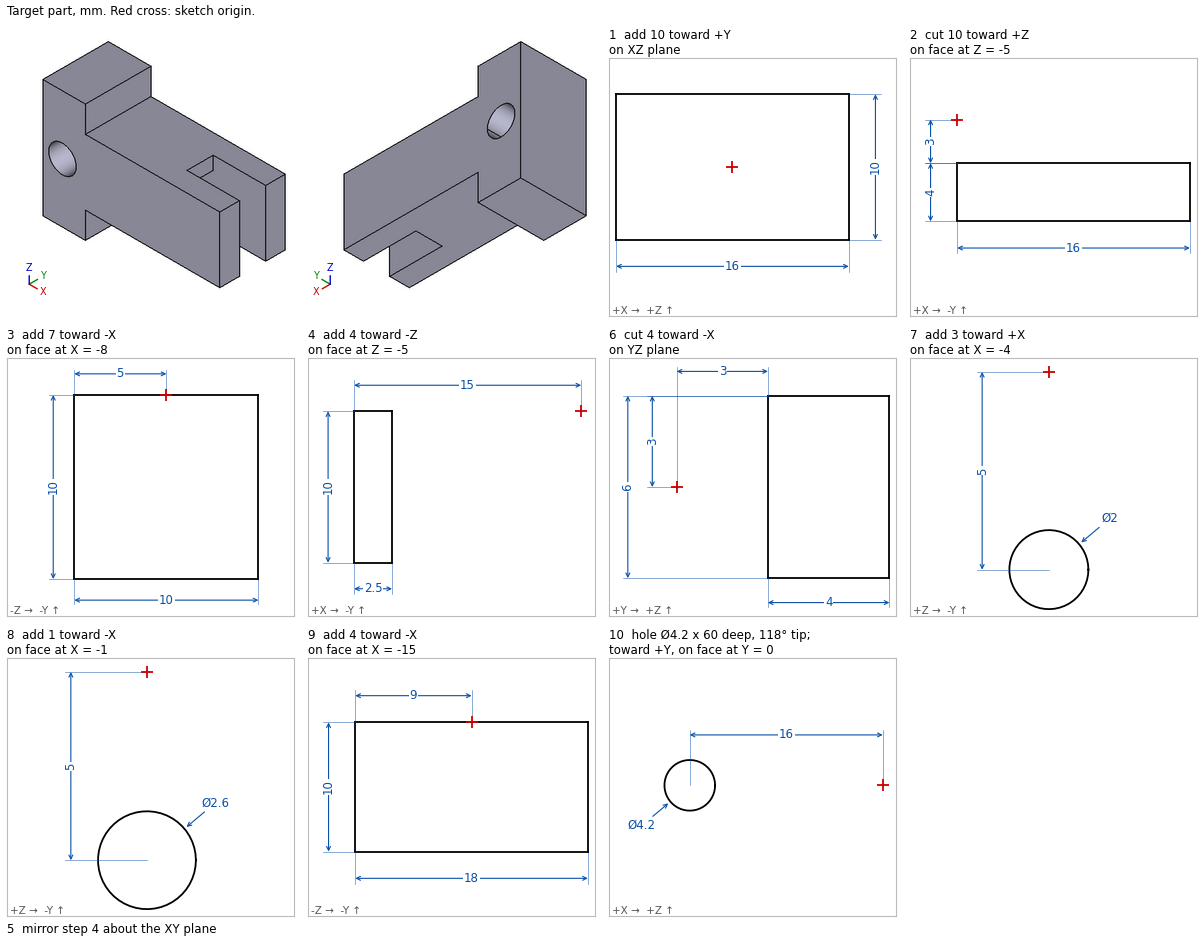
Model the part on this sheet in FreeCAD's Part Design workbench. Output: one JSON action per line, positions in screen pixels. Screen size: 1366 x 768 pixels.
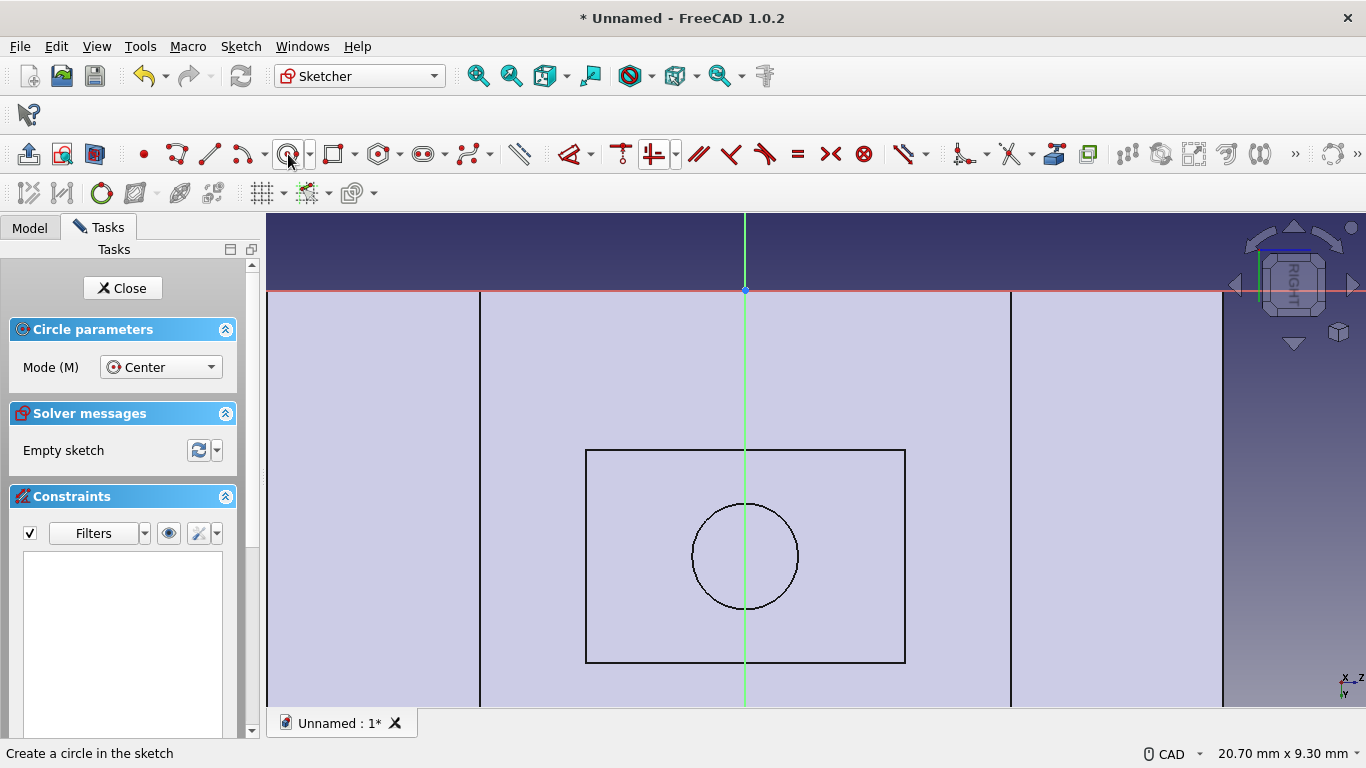
{"action": "left_click", "coordinate": [745, 556]}
{"action": "left_click", "coordinate": [794, 508]}
{"action": "key", "text": "Escape"}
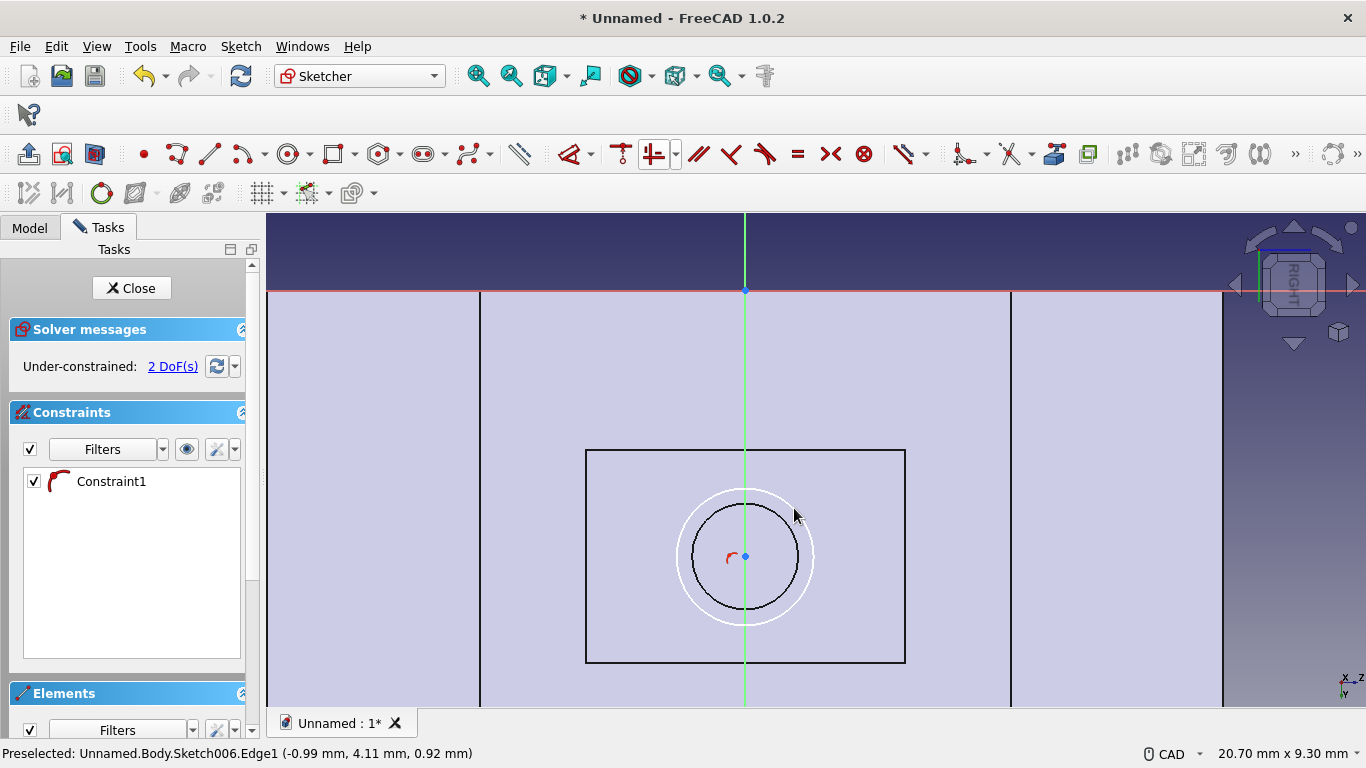
{"action": "left_click", "coordinate": [568, 154]}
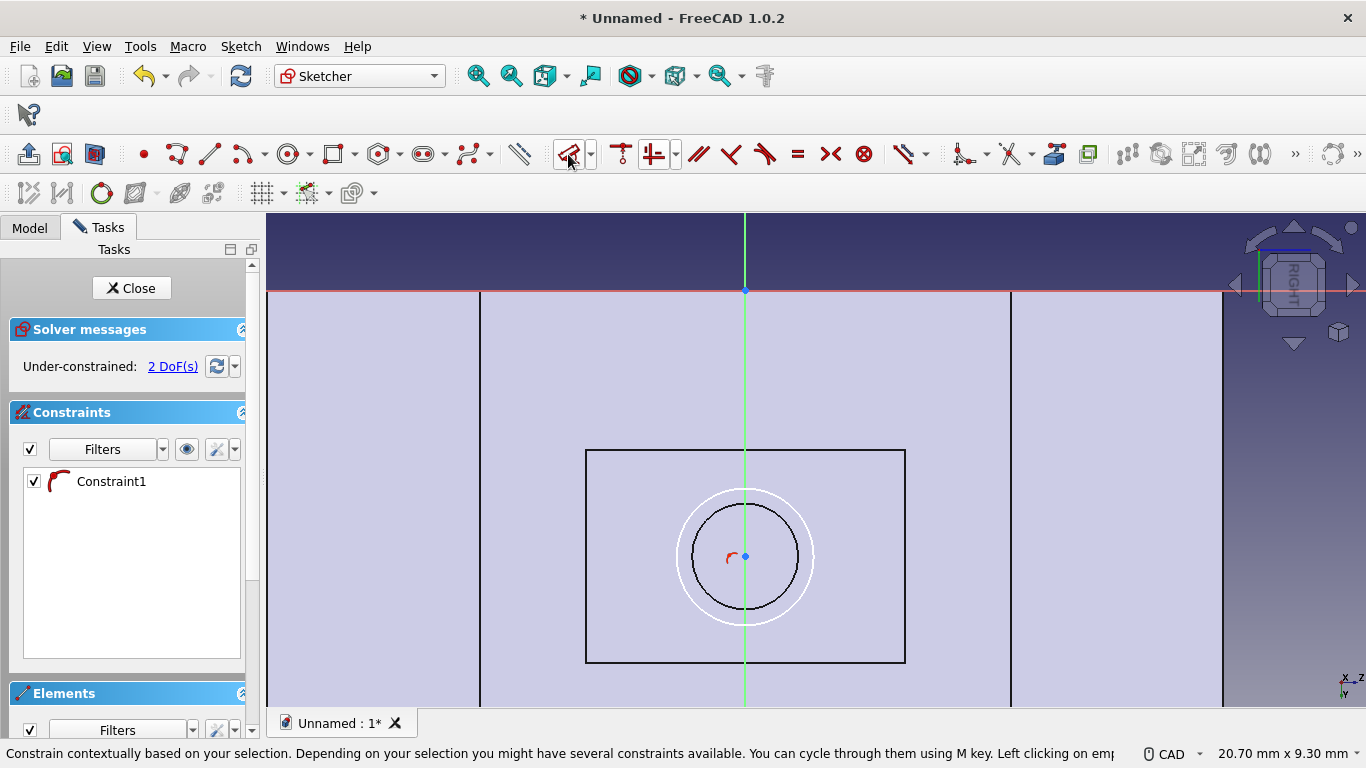
{"action": "left_click", "coordinate": [793, 508]}
{"action": "left_click", "coordinate": [815, 485]}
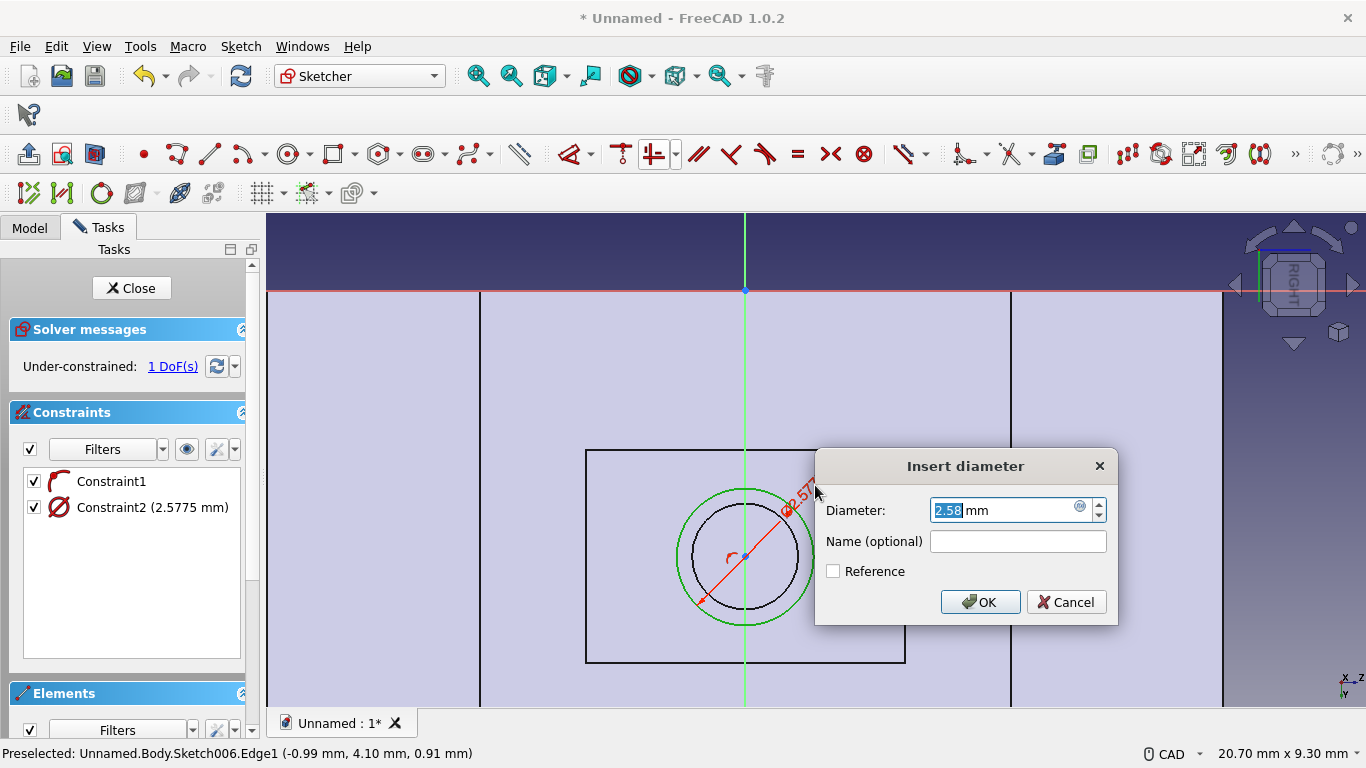
{"action": "type", "text": "2.6"}
{"action": "key", "text": "Return"}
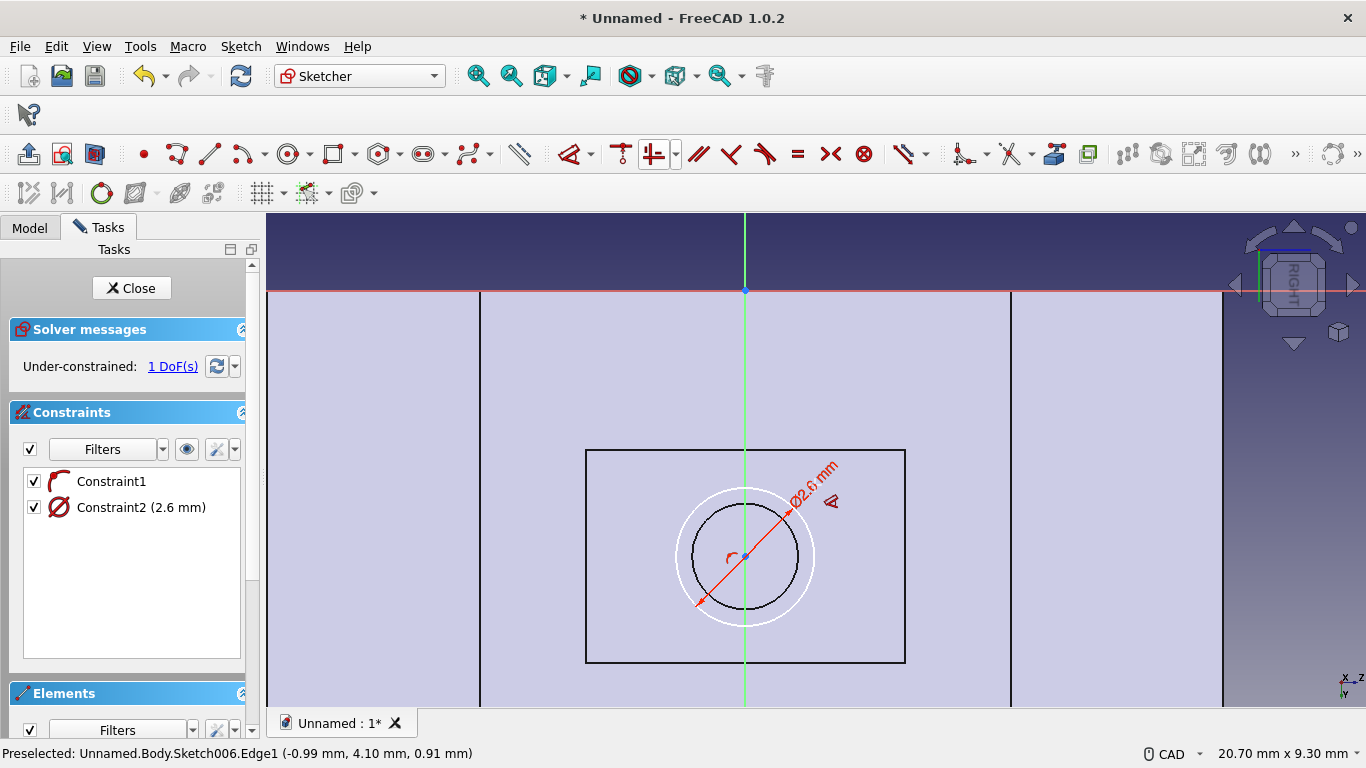
{"action": "left_click", "coordinate": [745, 557]}
{"action": "left_click", "coordinate": [779, 424]}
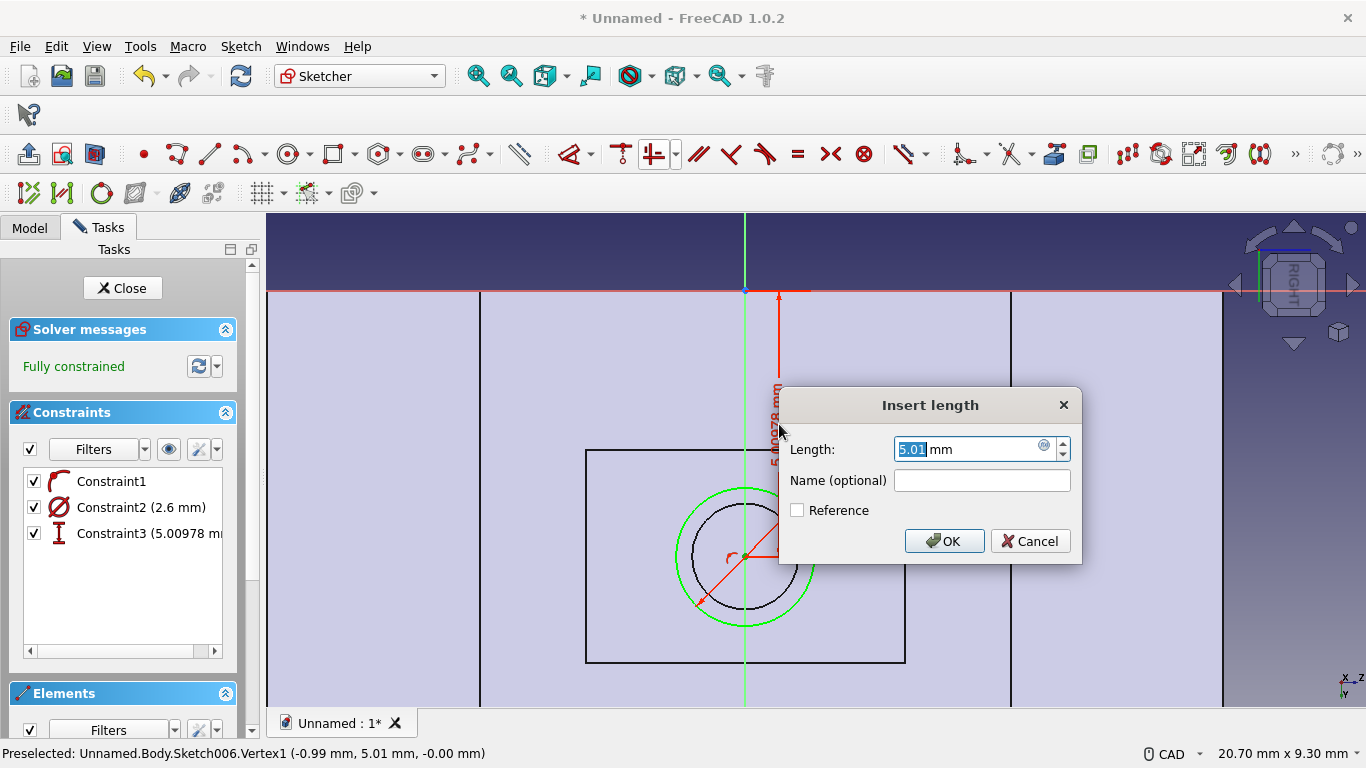
{"action": "type", "text": "5"}
{"action": "key", "text": "Return"}
{"action": "key", "text": "Escape"}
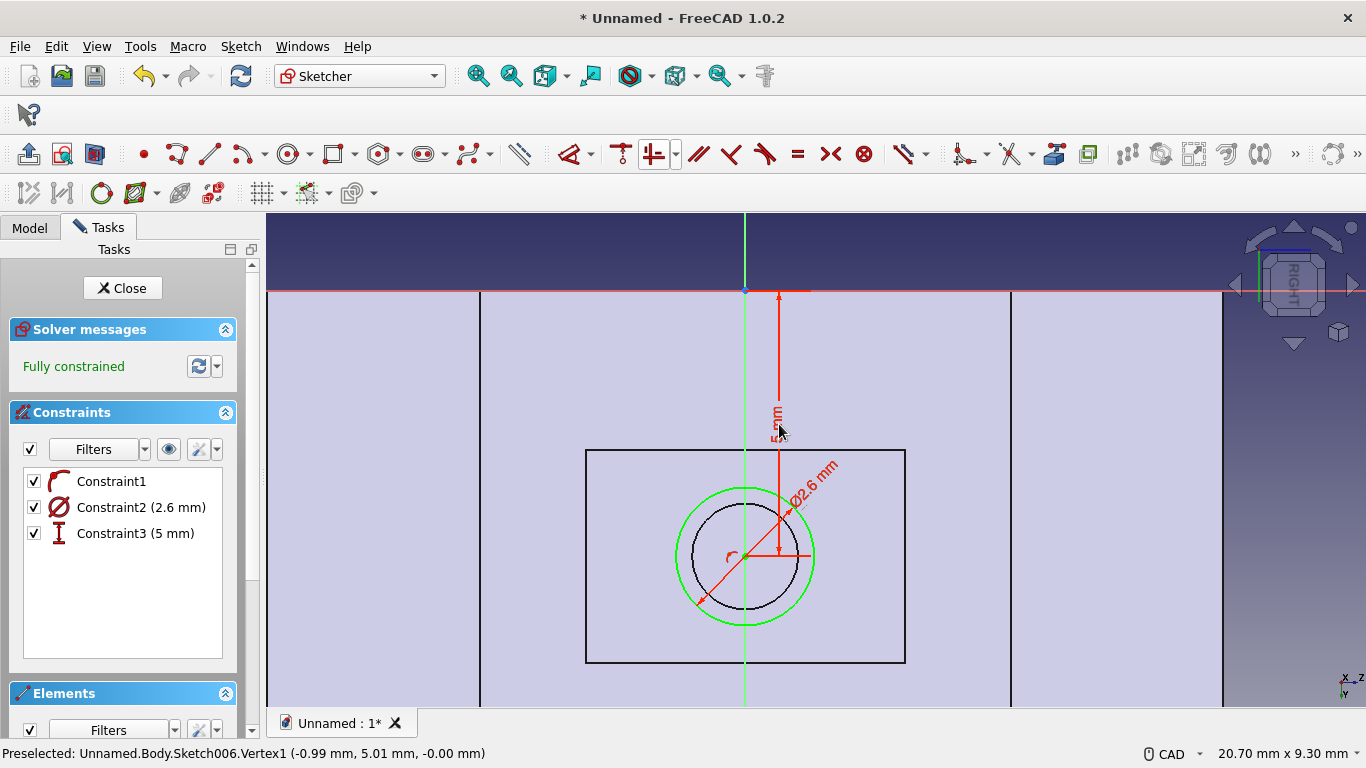
{"action": "left_click", "coordinate": [123, 288]}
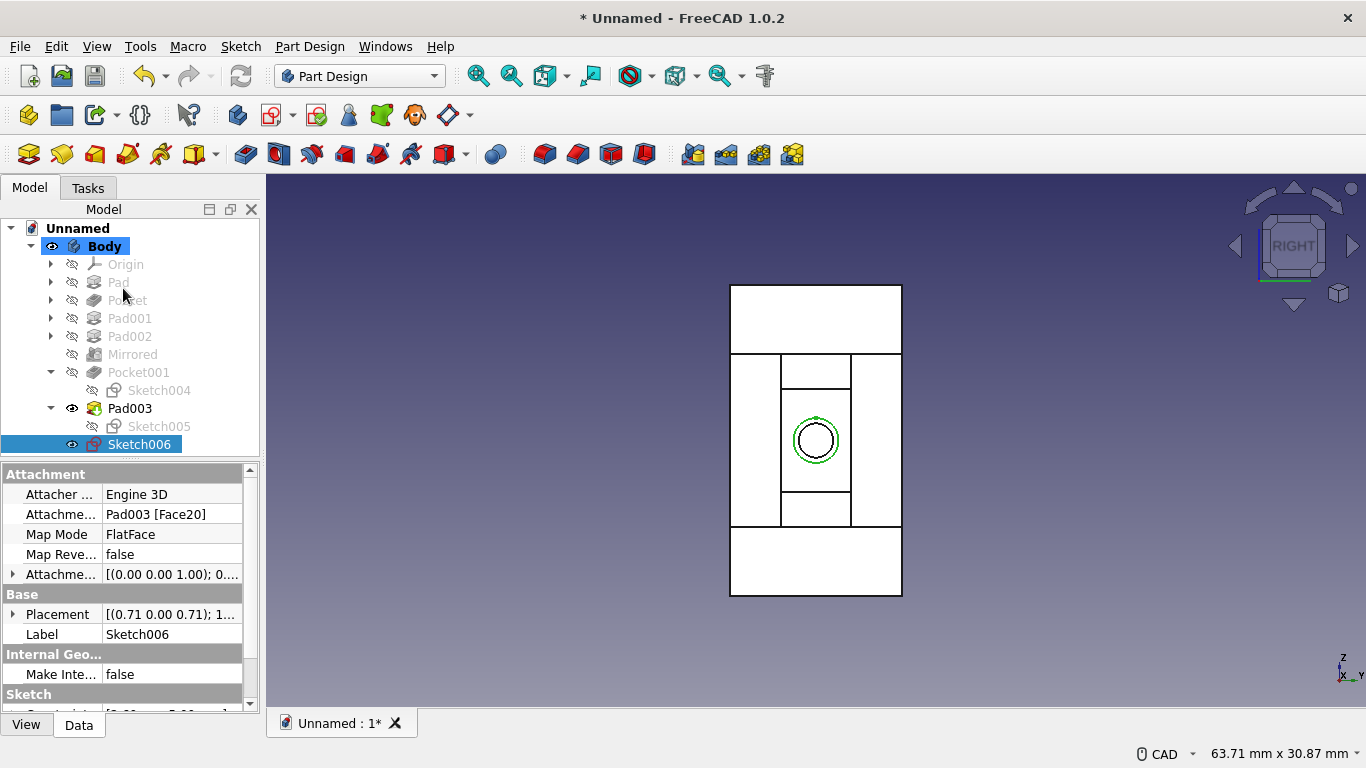
{"action": "left_click", "coordinate": [29, 154]}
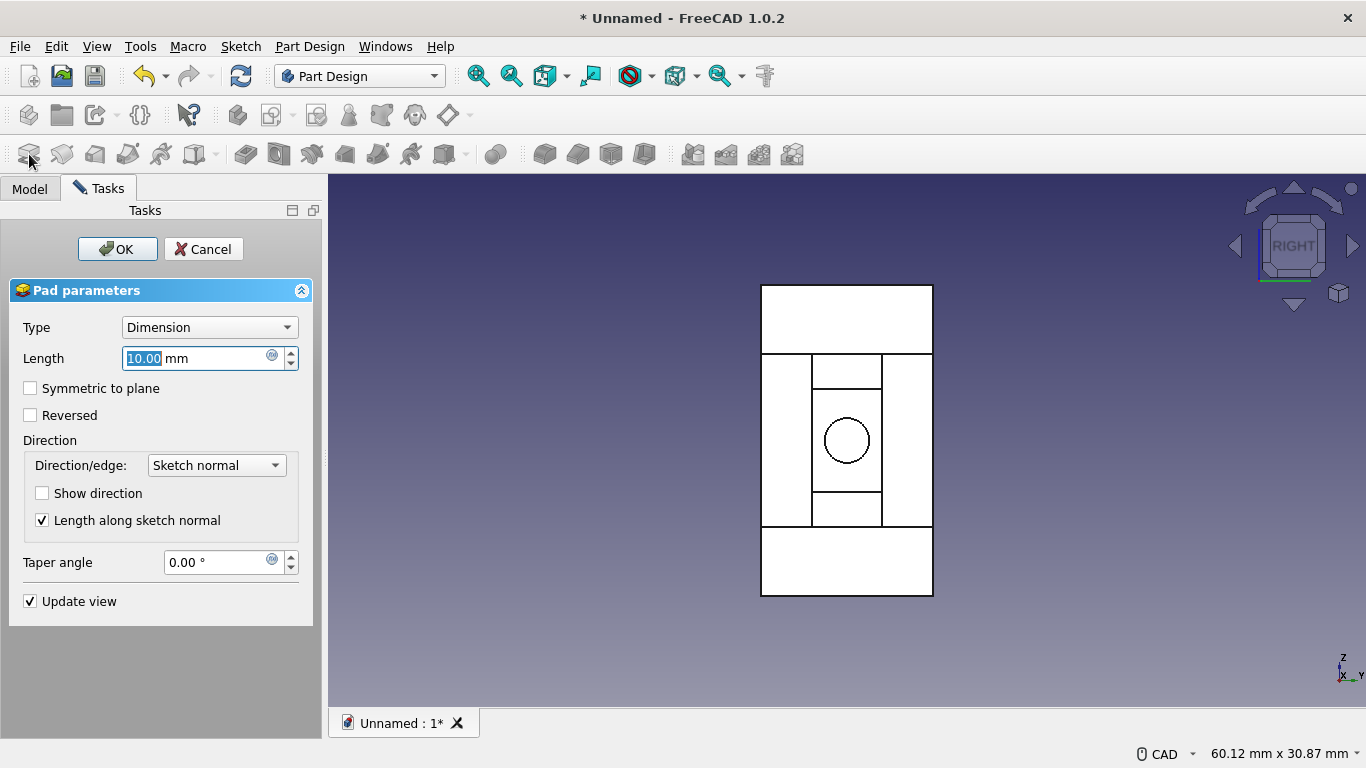
{"action": "type", "text": "1"}
{"action": "key", "text": "Tab"}